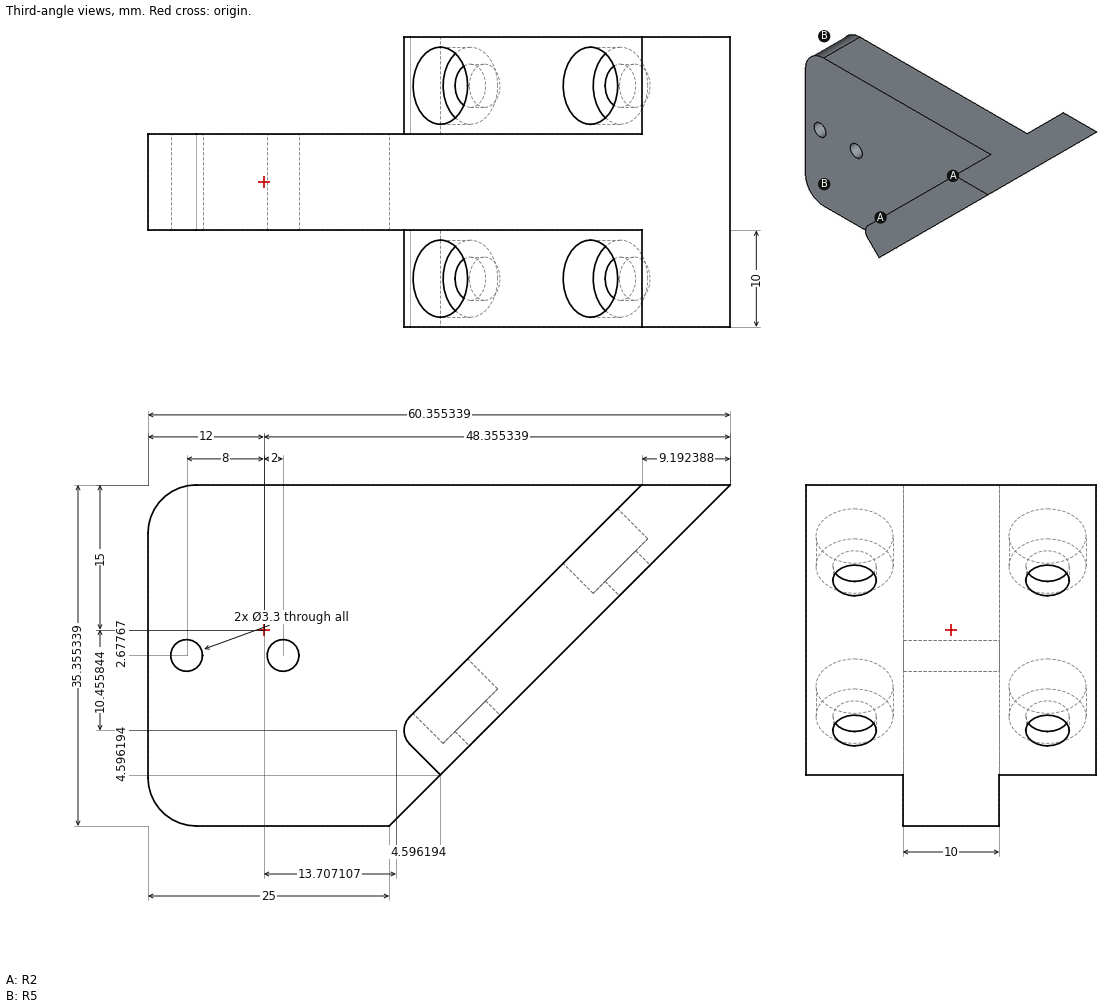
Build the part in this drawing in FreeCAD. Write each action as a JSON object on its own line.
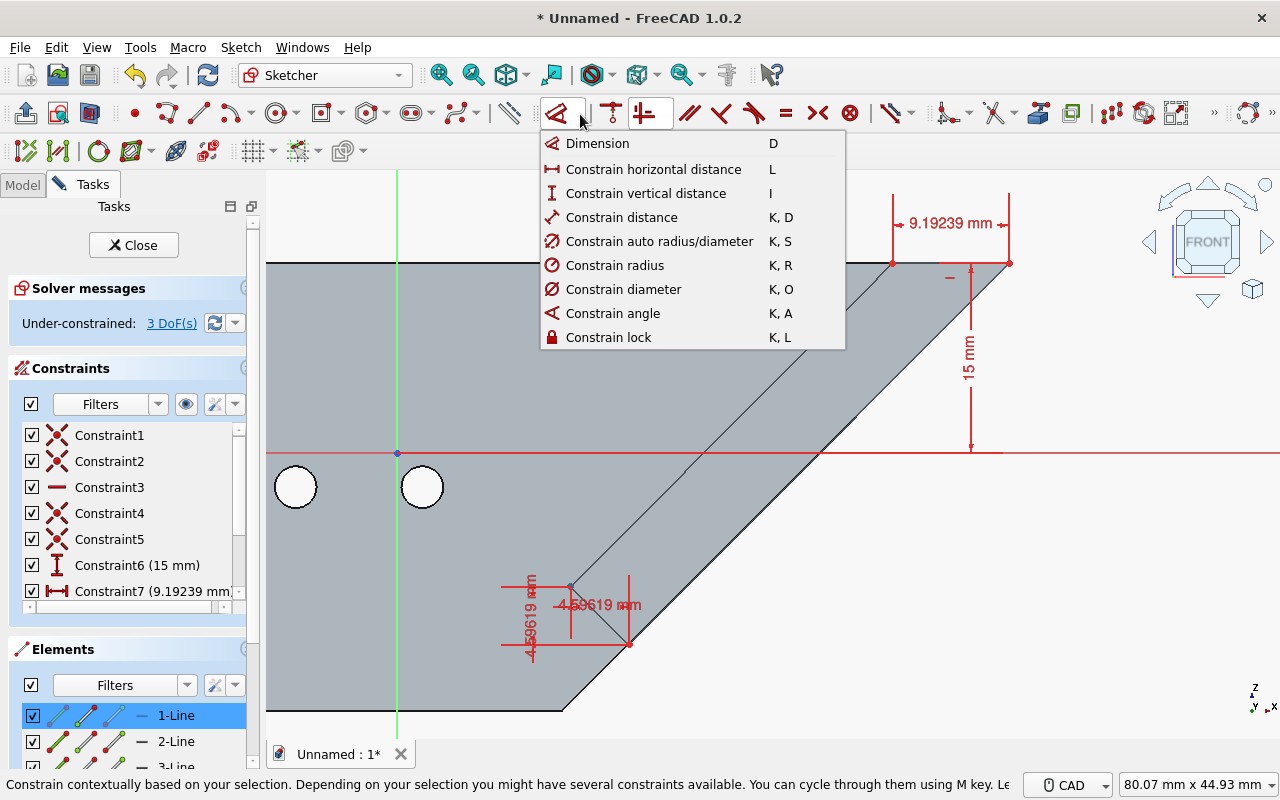
{"action": "left_click", "coordinate": [693, 169]}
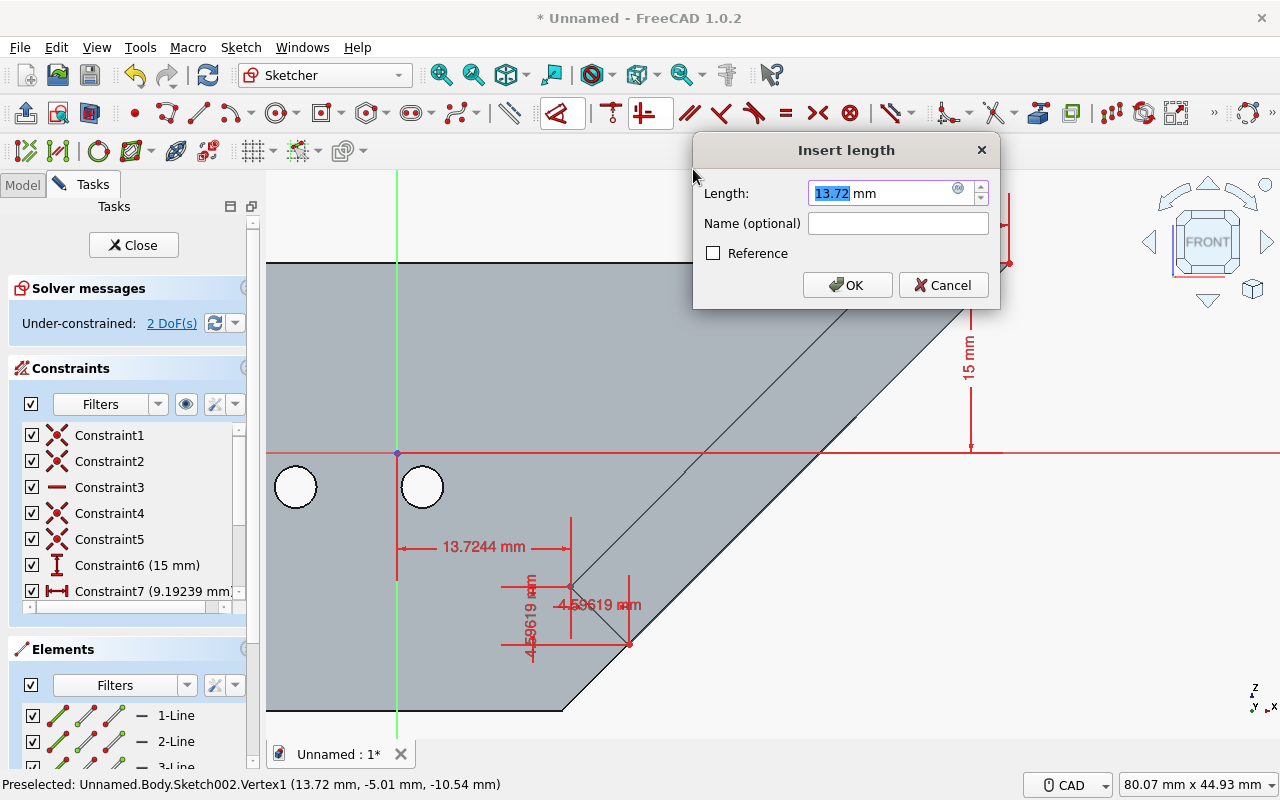
{"action": "type", "text": "13.707107"}
{"action": "key", "text": "Return"}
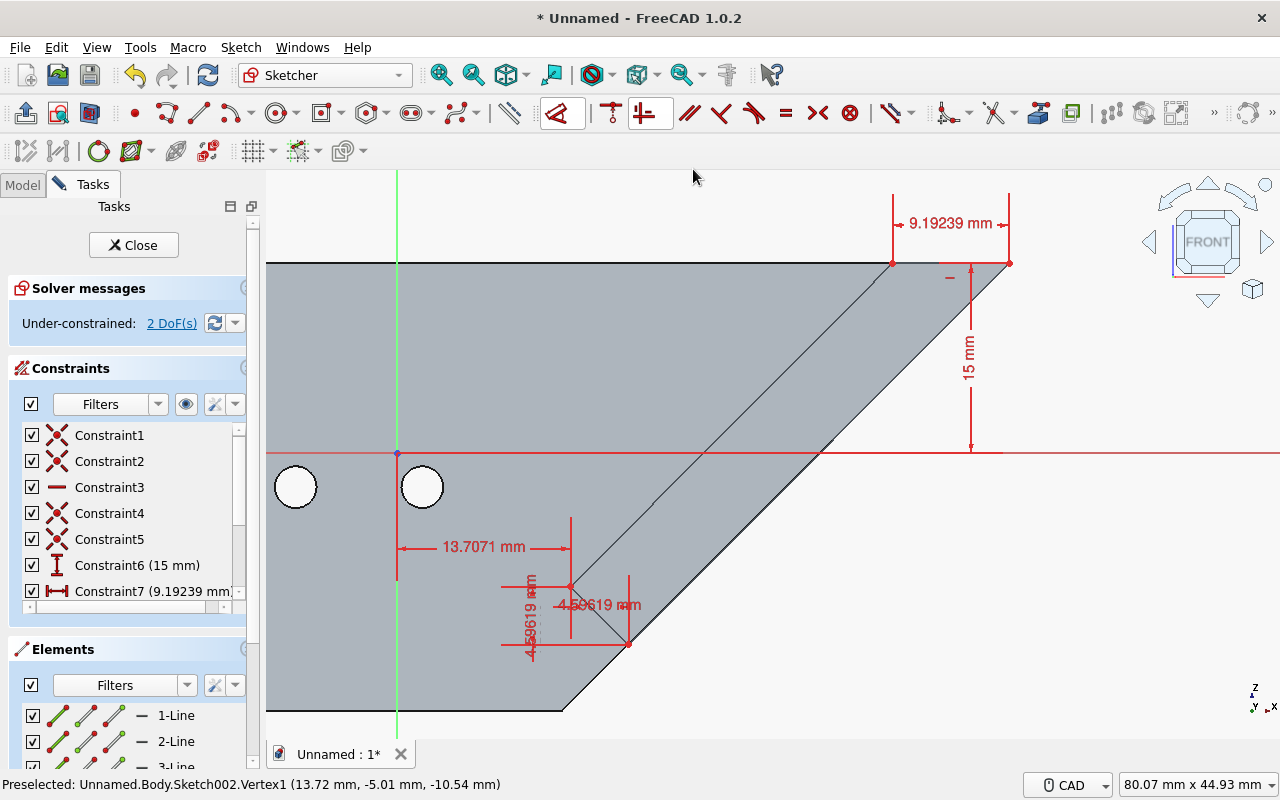
{"action": "left_click", "coordinate": [571, 587]}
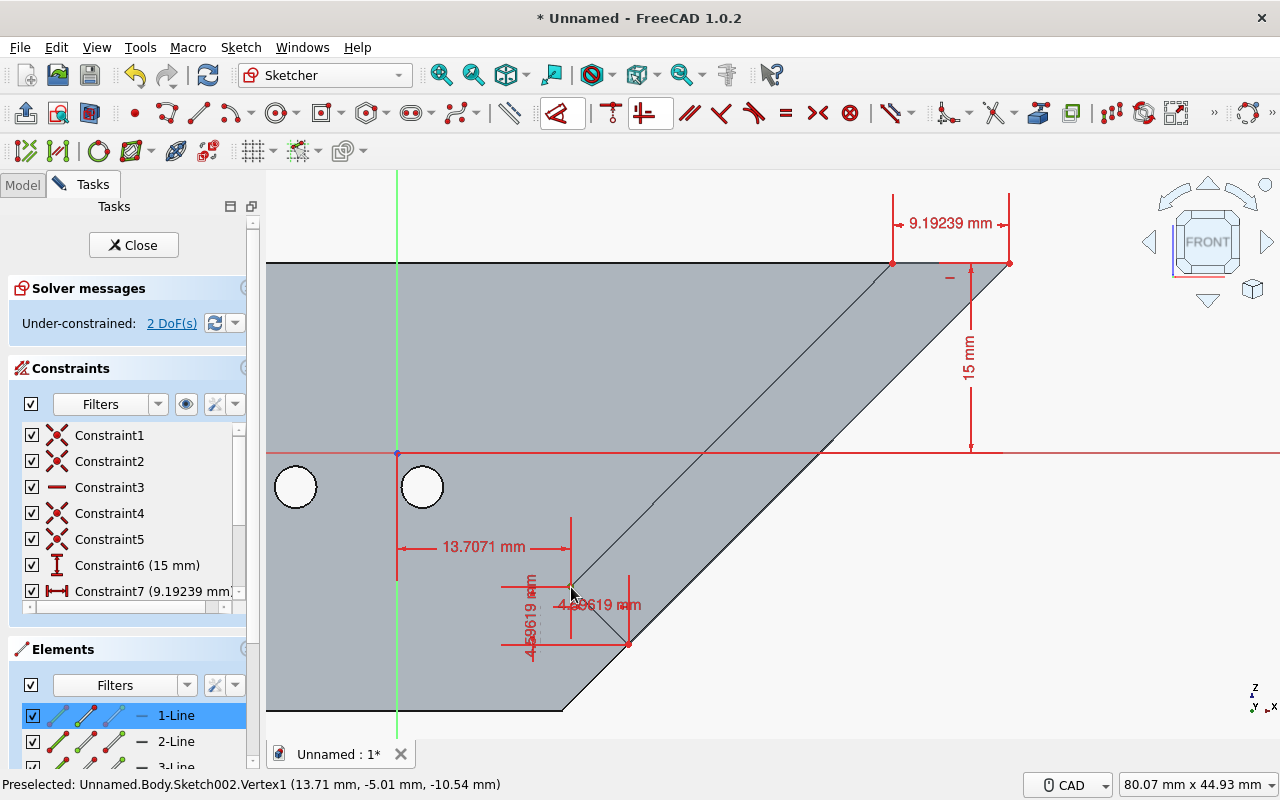
{"action": "key", "text": "i"}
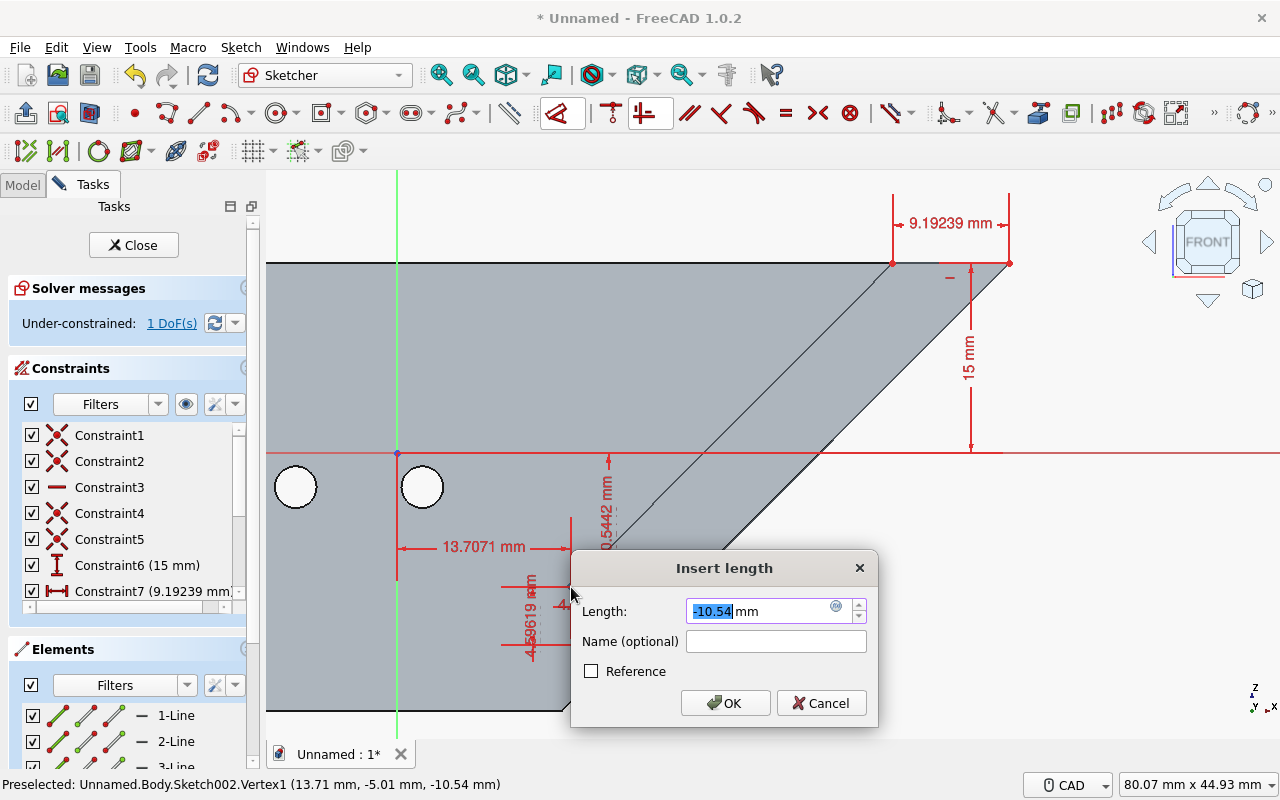
{"action": "type", "text": "-10.455844"}
{"action": "key", "text": "Return"}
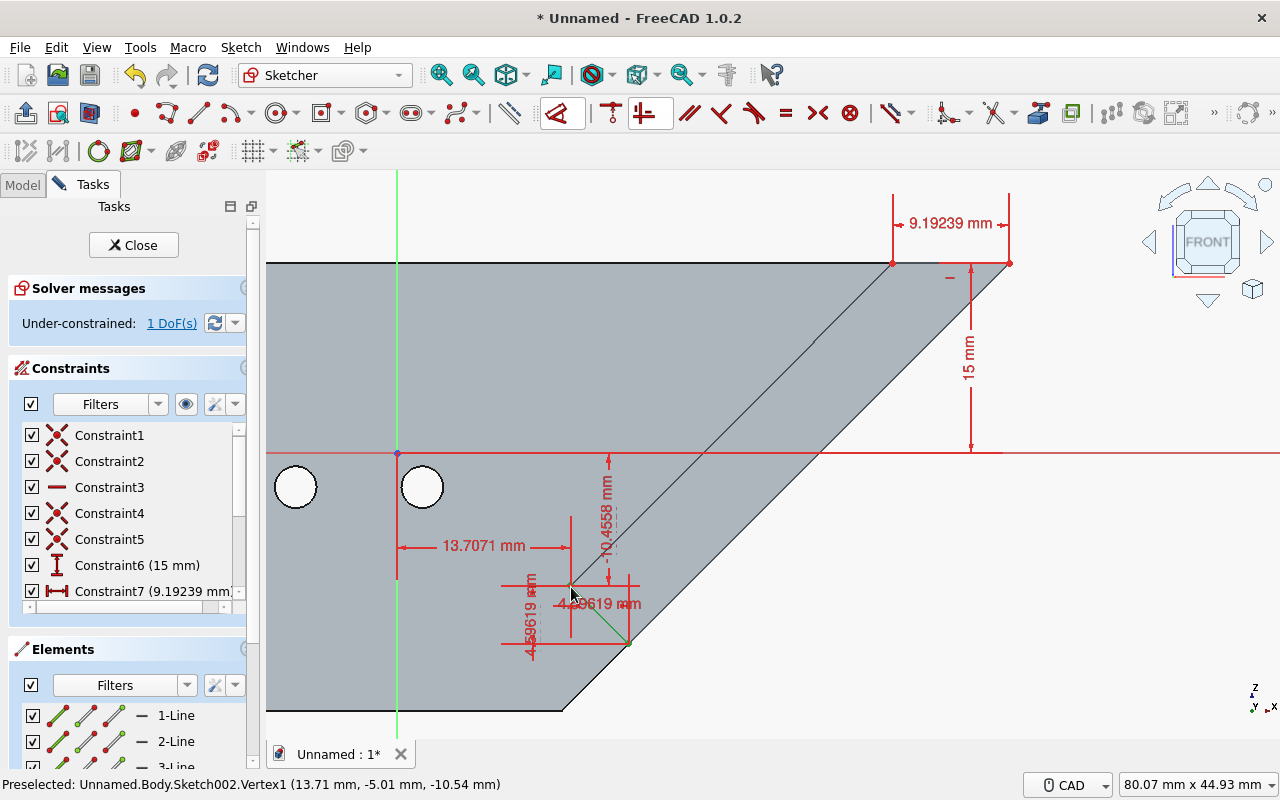
{"action": "left_click", "coordinate": [1009, 263]}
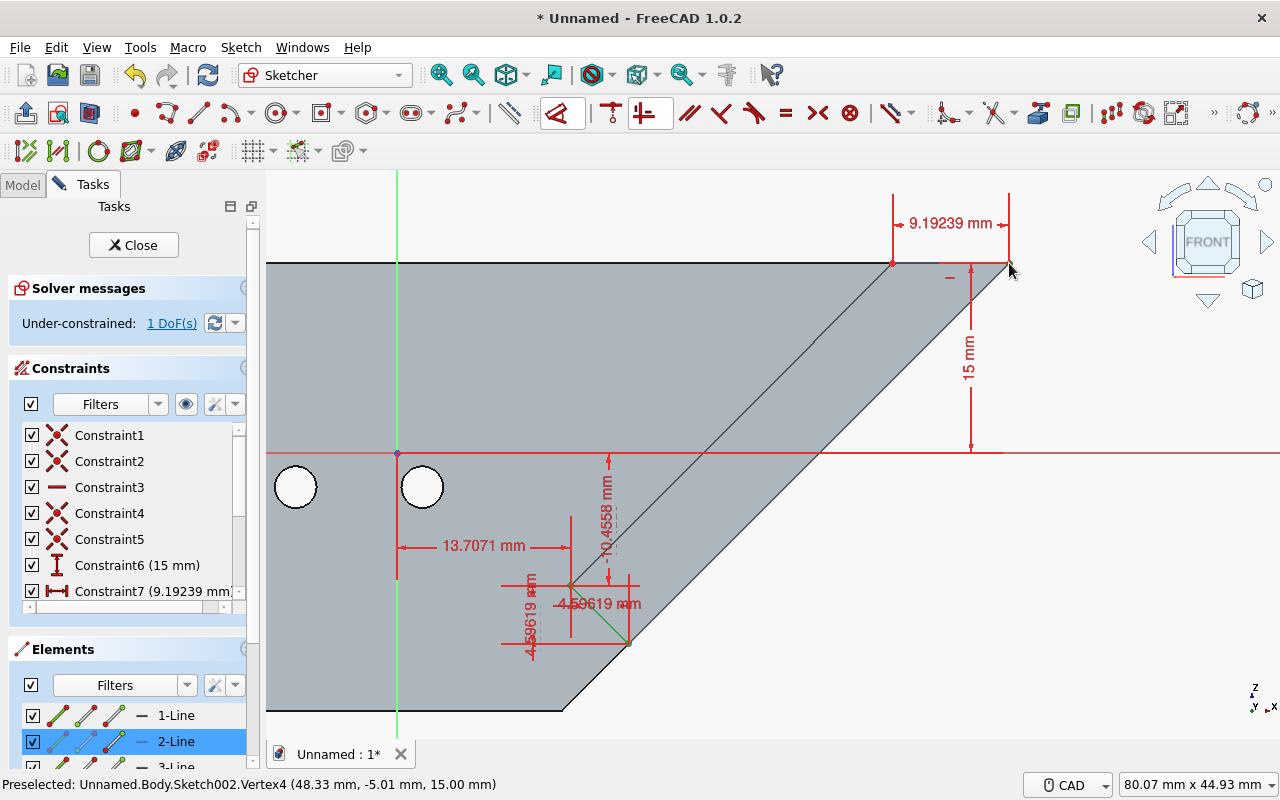
{"action": "left_click", "coordinate": [580, 114]}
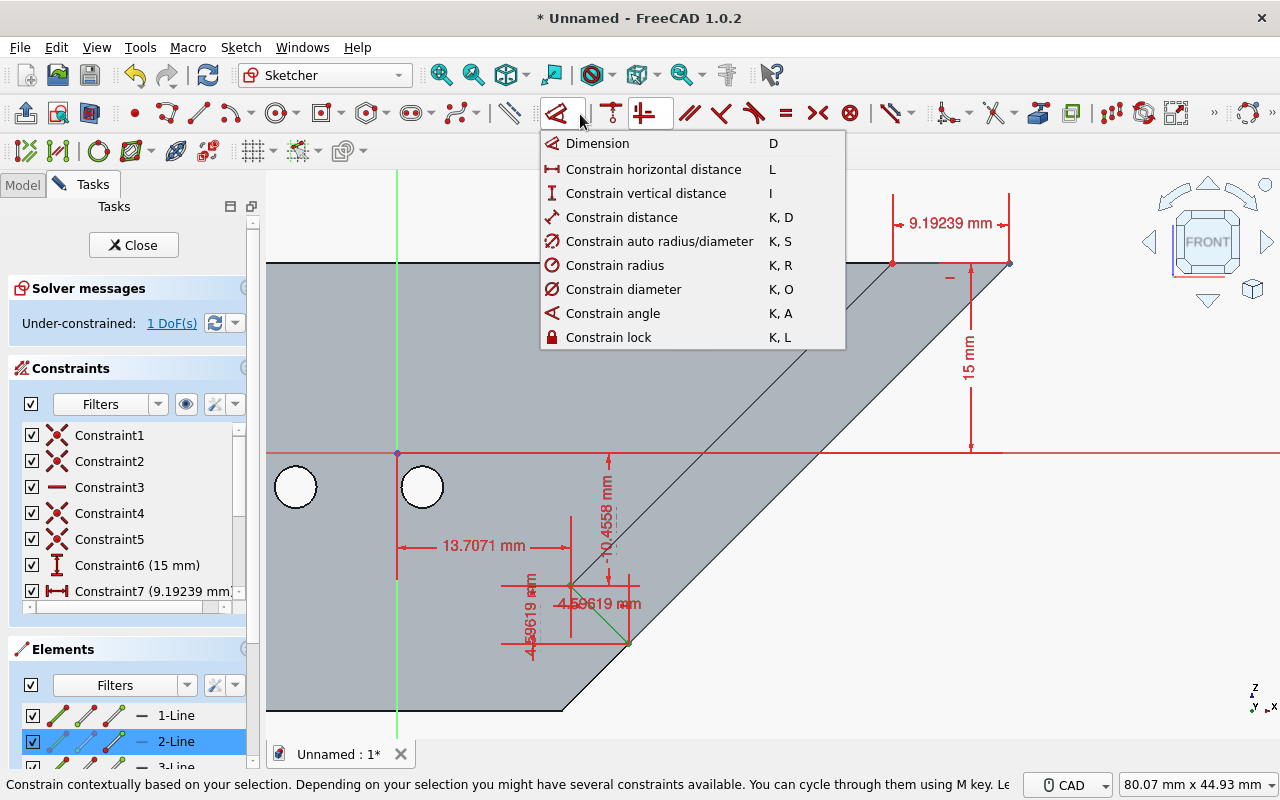
{"action": "left_click", "coordinate": [693, 169]}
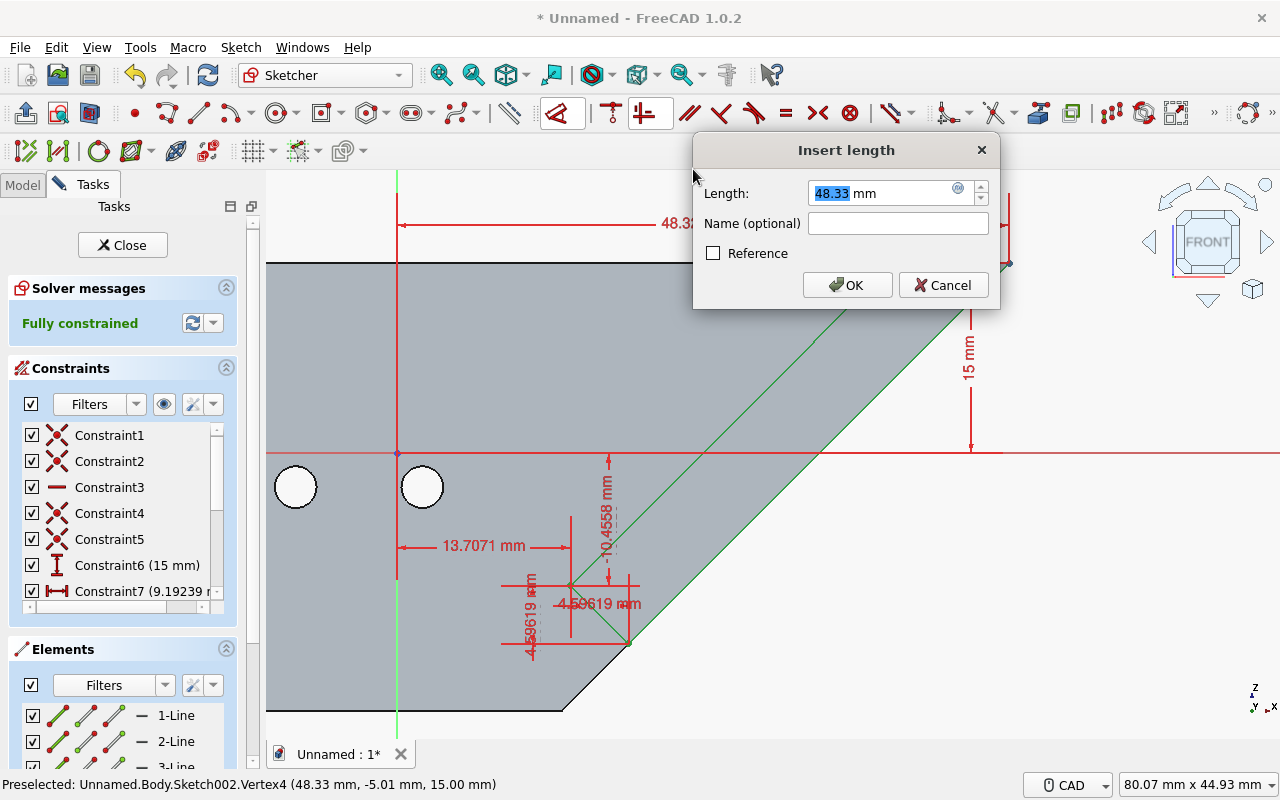
{"action": "type", "text": "48.355339"}
{"action": "key", "text": "Return"}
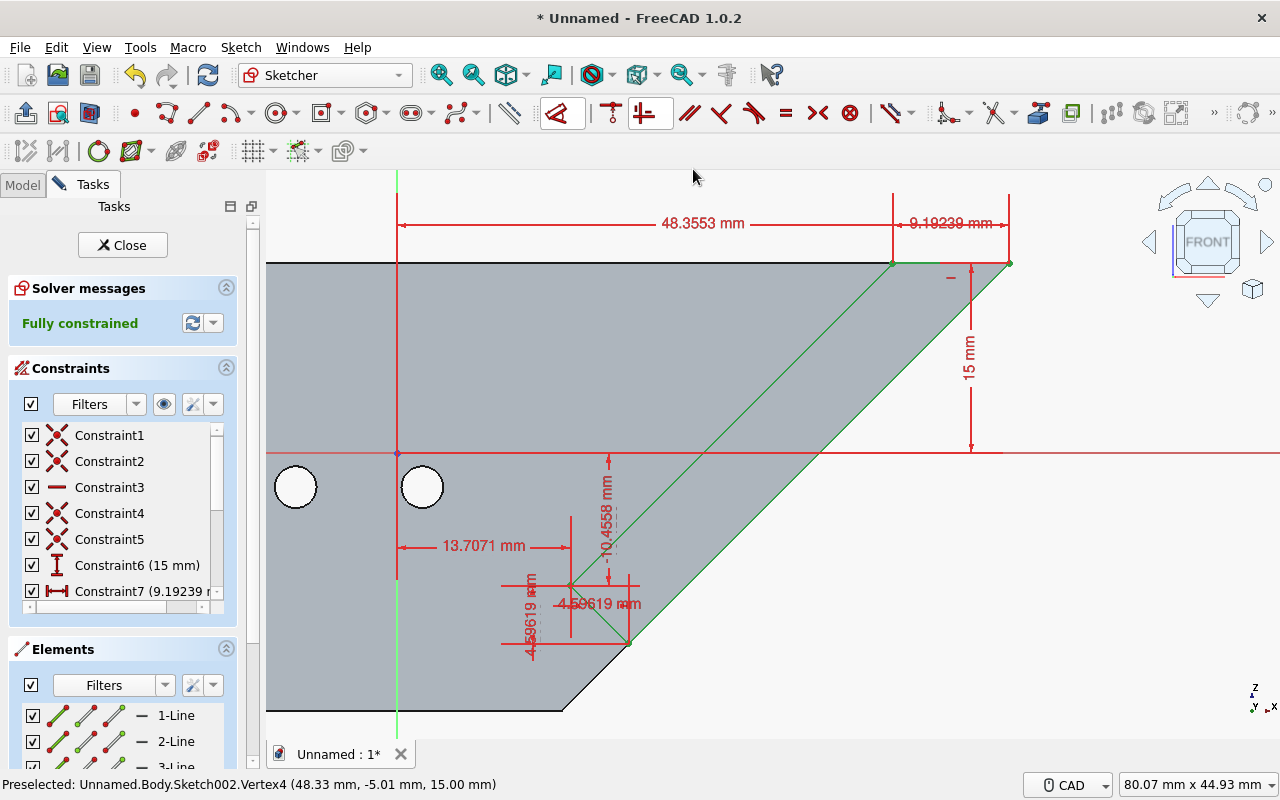
{"action": "left_click", "coordinate": [123, 245]}